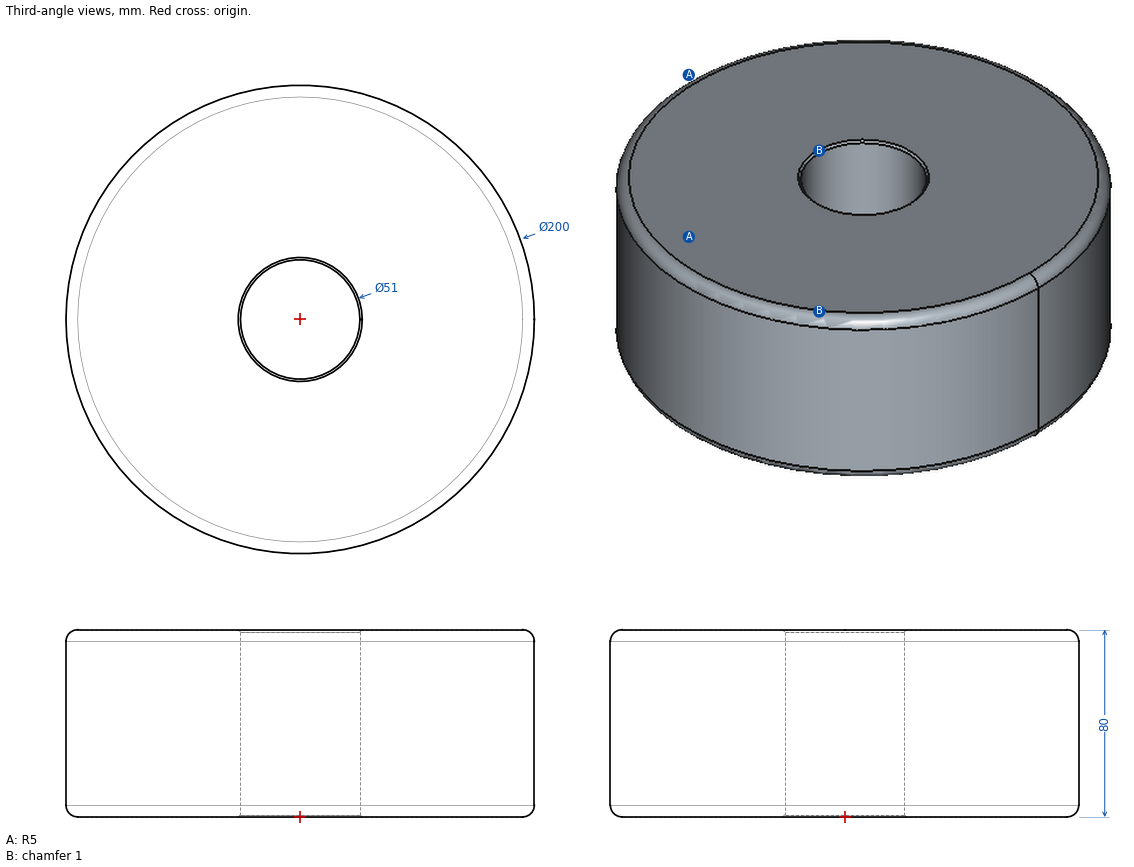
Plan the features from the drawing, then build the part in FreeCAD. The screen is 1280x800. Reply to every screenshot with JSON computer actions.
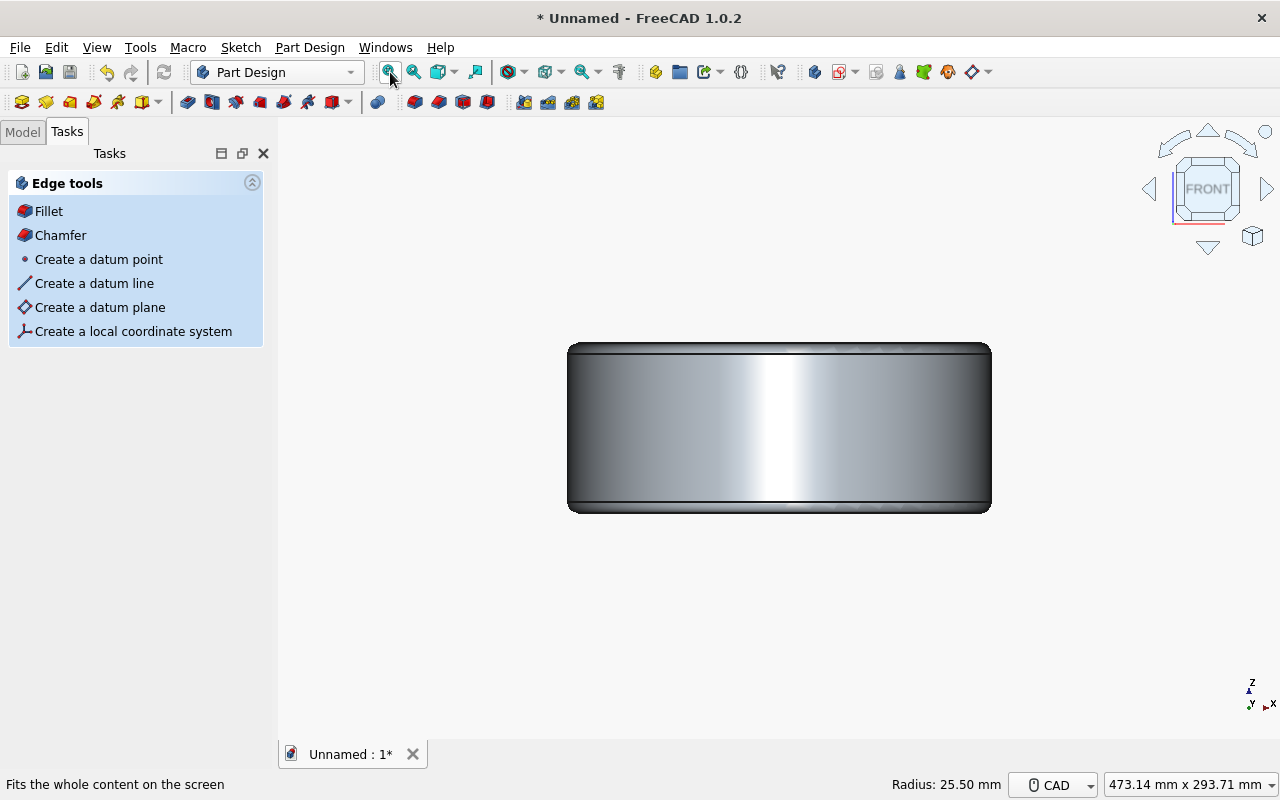
{"action": "key", "text": "3"}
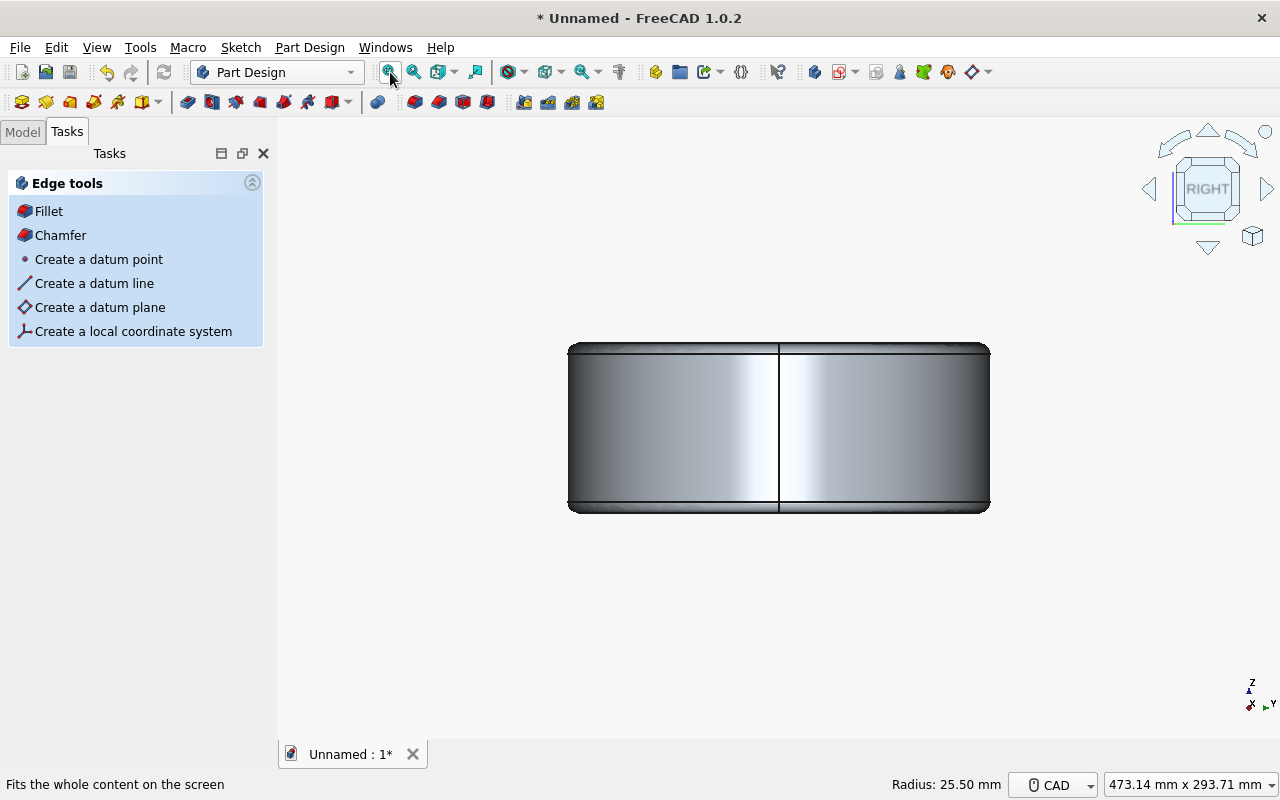
{"action": "left_click", "coordinate": [390, 72]}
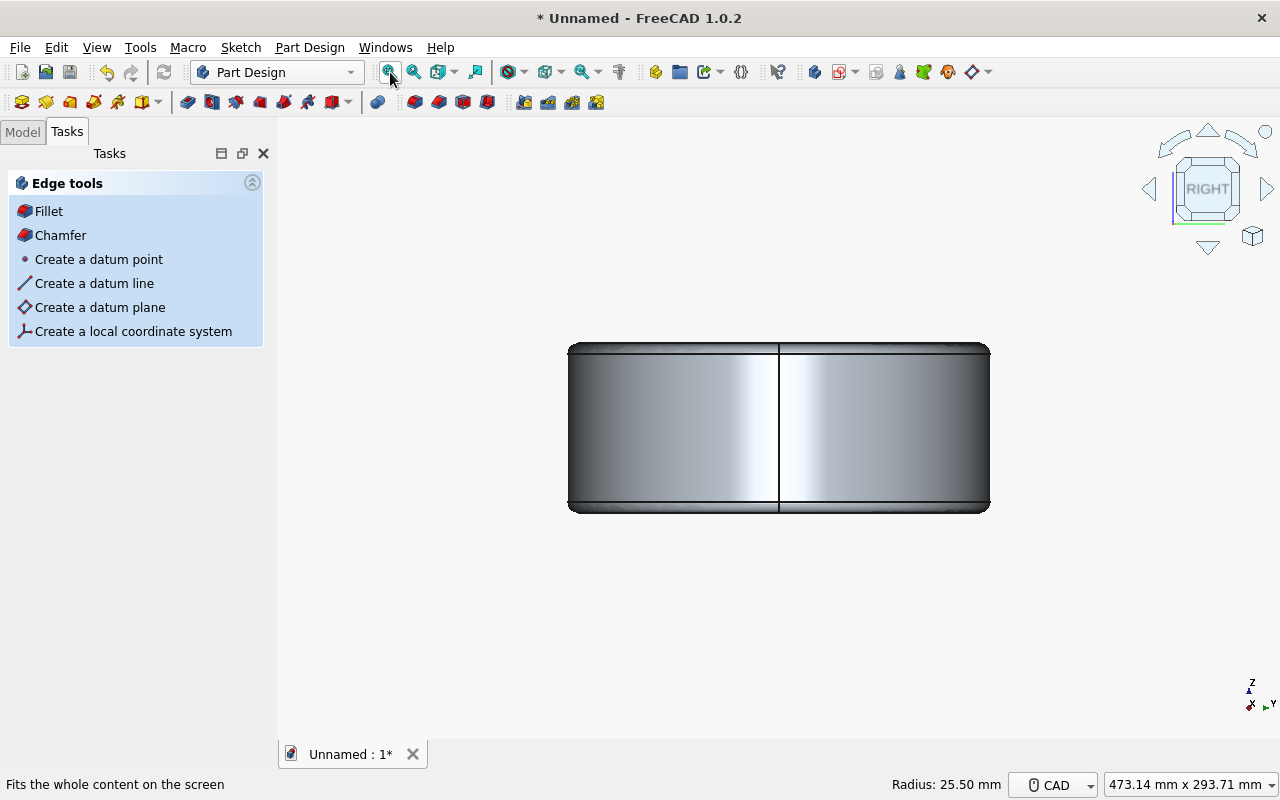
{"action": "key", "text": "5"}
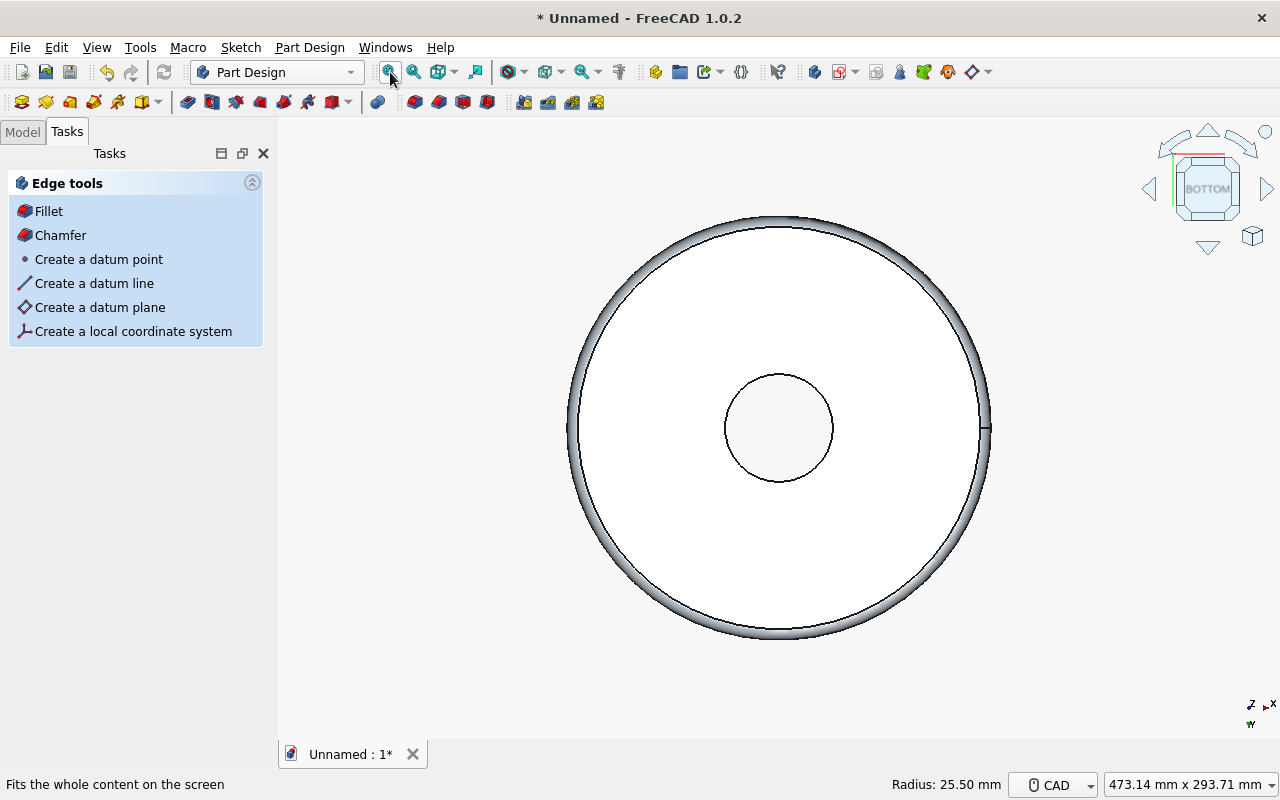
{"action": "left_click", "coordinate": [725, 427], "text": "ctrl"}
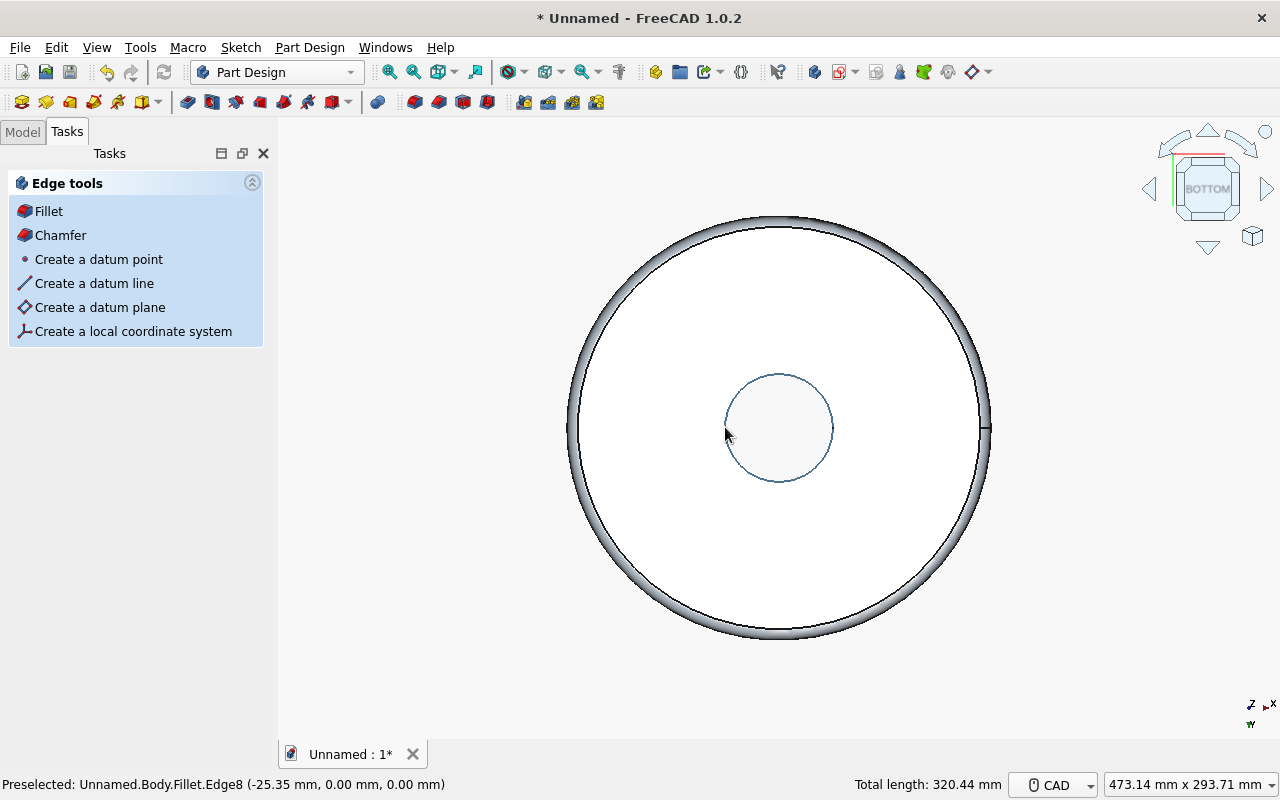
{"action": "left_click", "coordinate": [440, 102]}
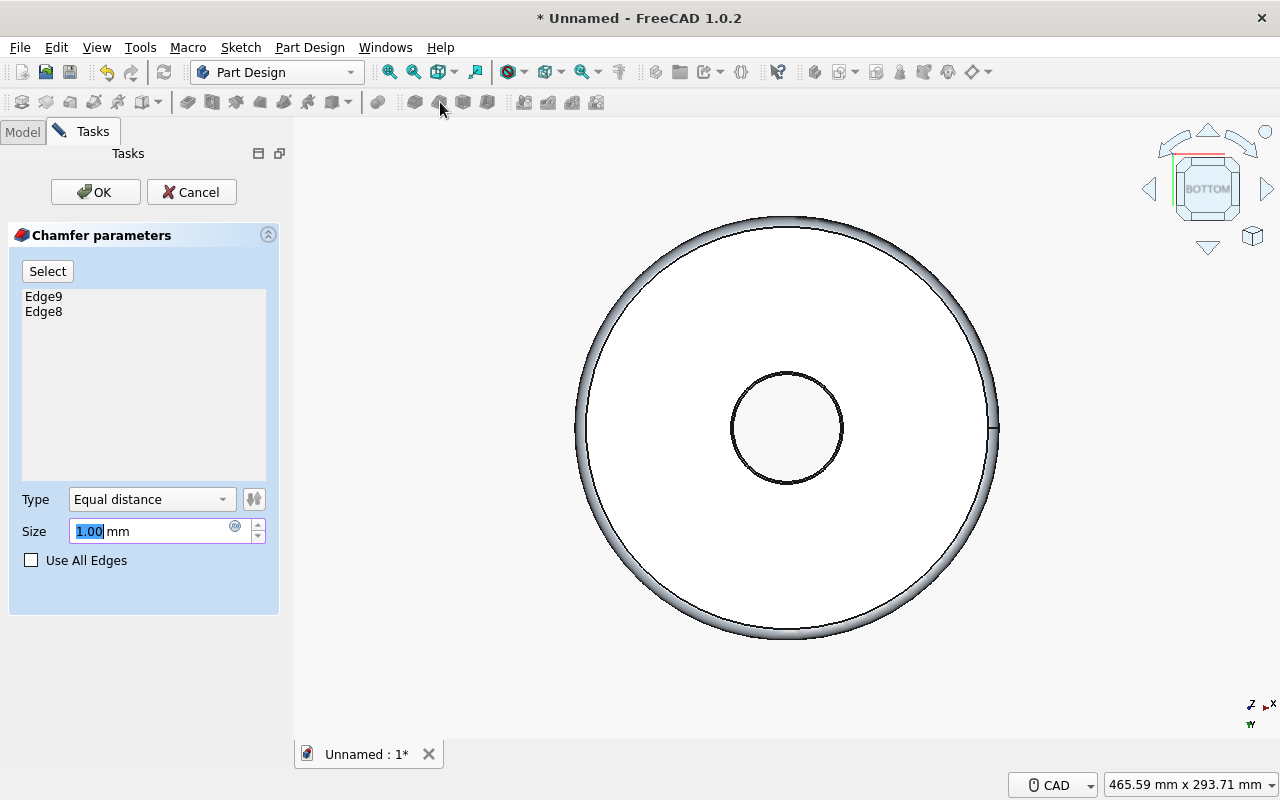
{"action": "type", "text": "1"}
{"action": "key", "text": "Tab"}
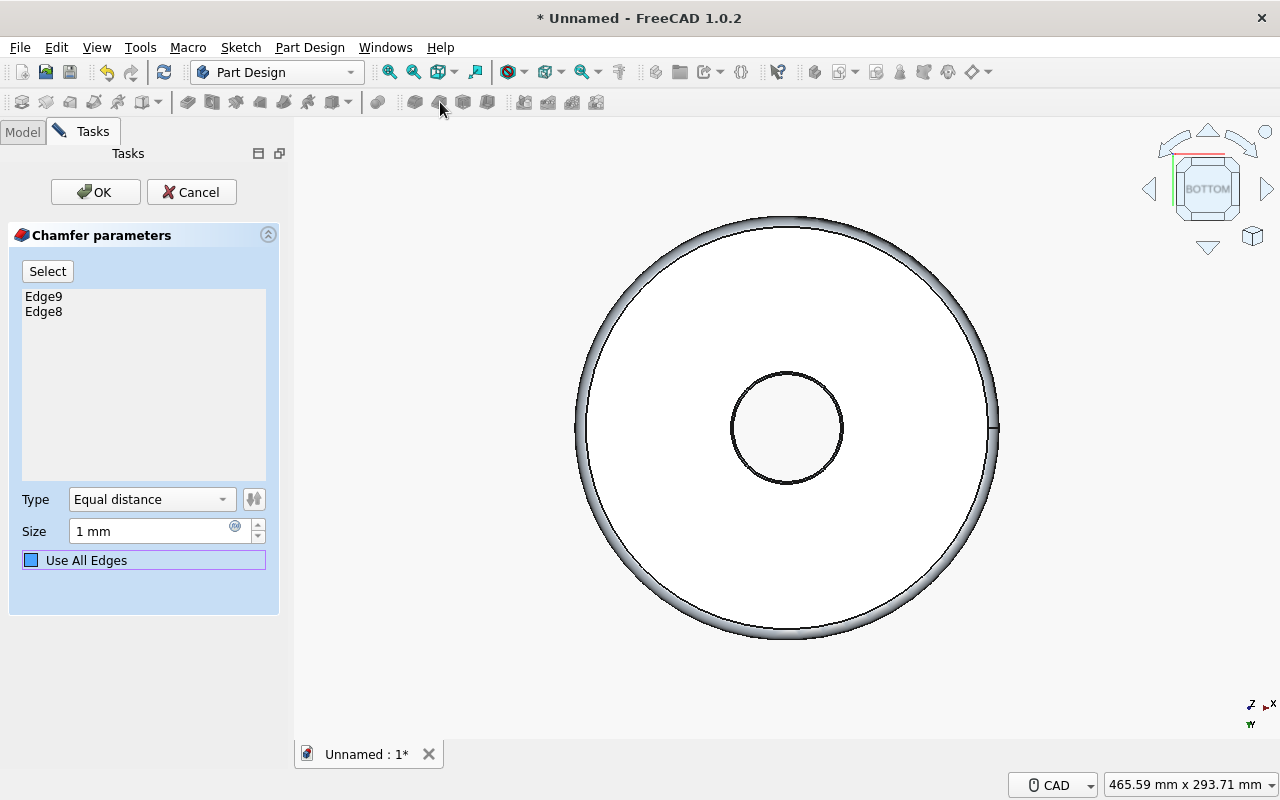
{"action": "left_click", "coordinate": [96, 192]}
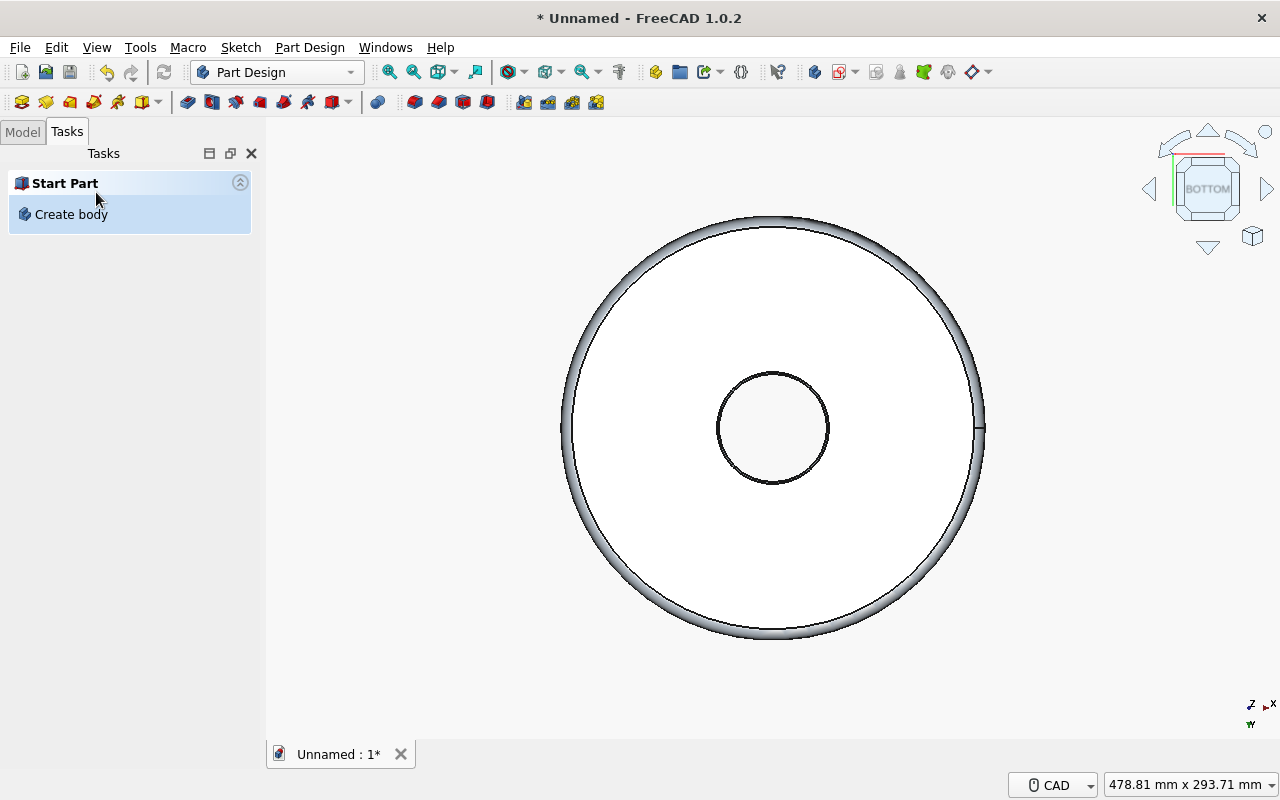
{"action": "key", "text": "0"}